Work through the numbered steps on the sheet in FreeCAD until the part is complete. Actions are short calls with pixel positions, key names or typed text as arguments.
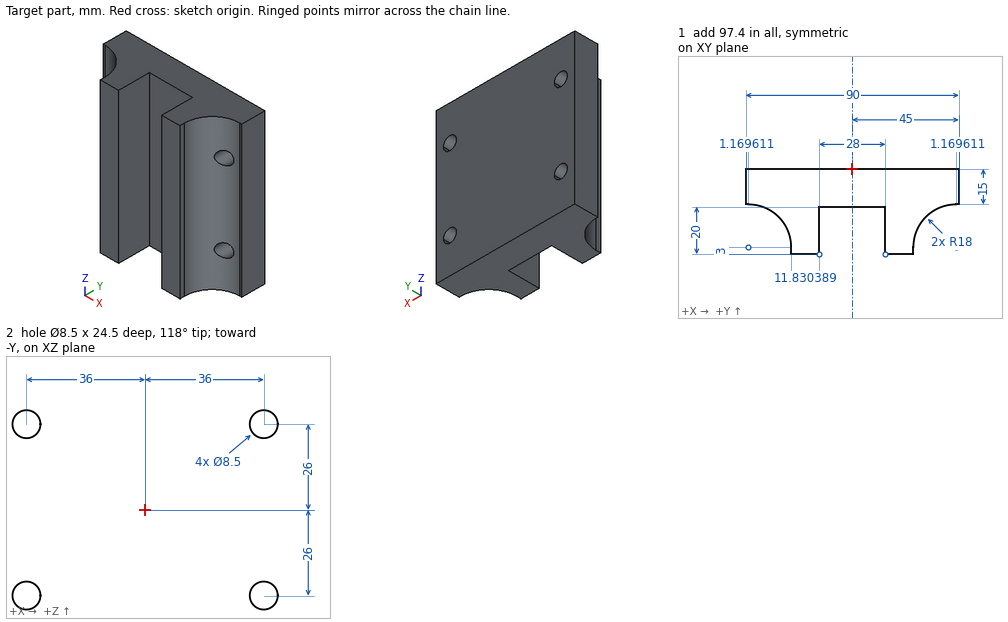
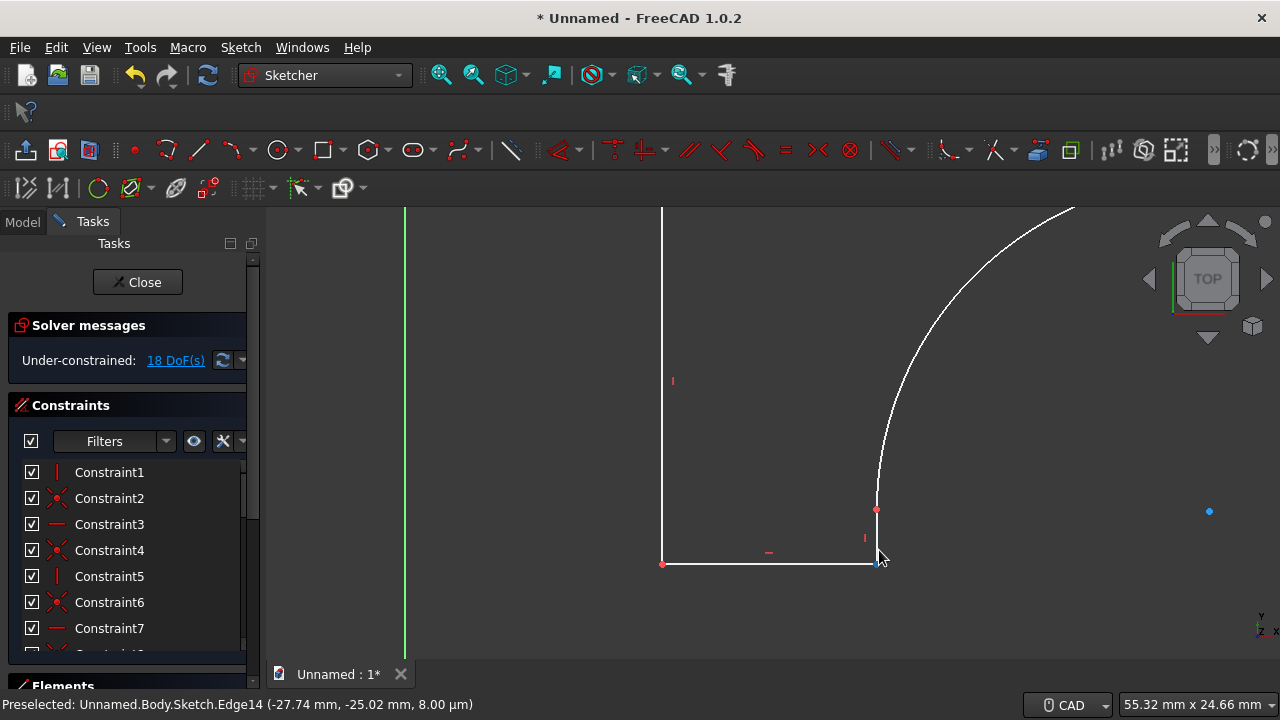
click(877, 548)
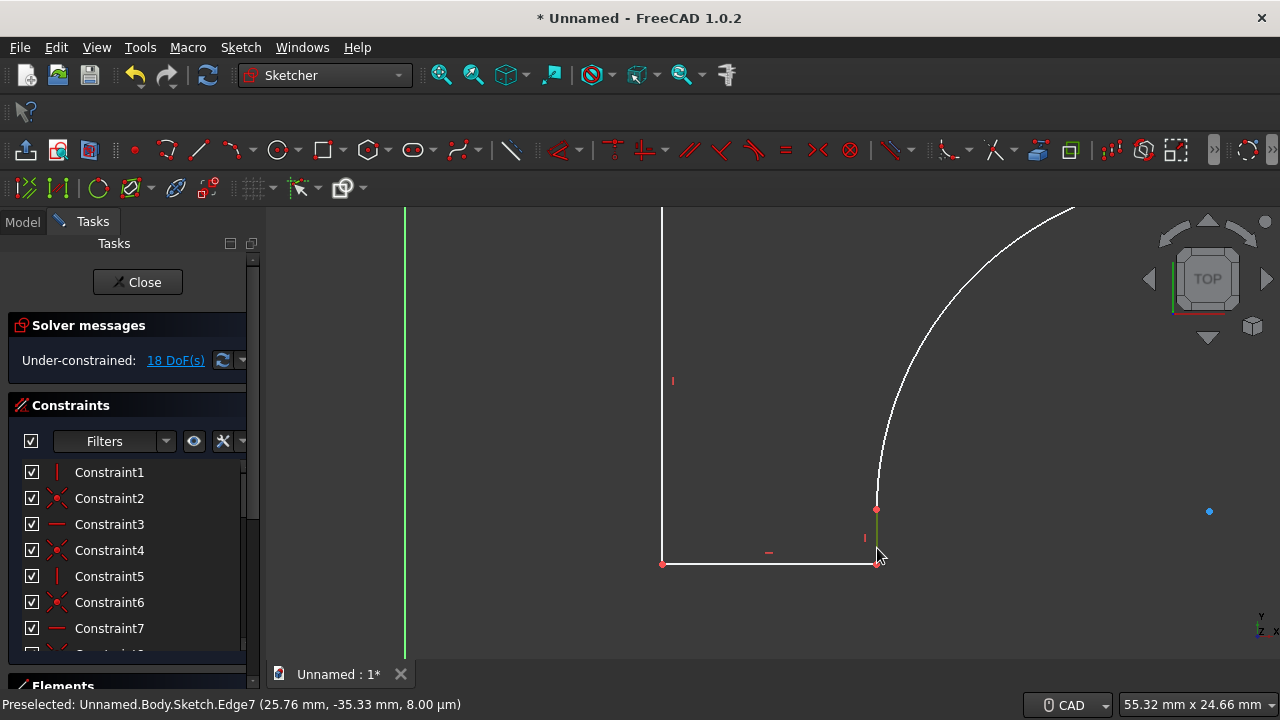
click(913, 360)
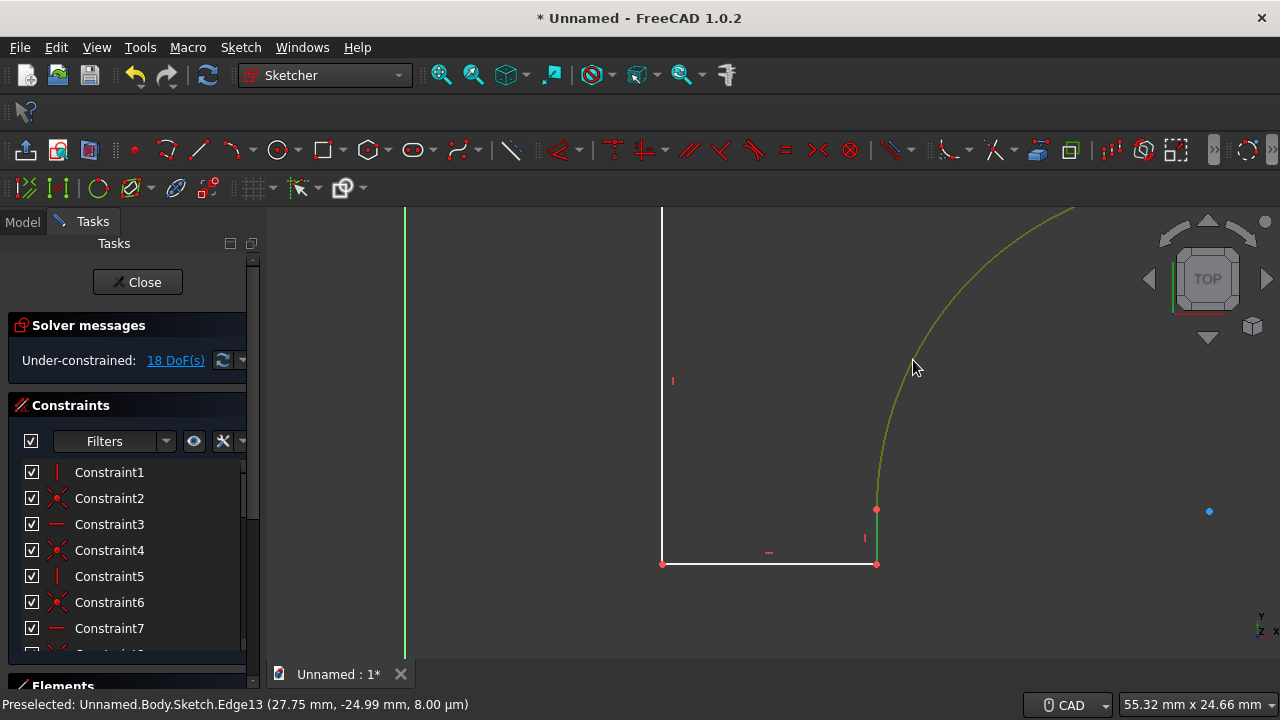
click(754, 150)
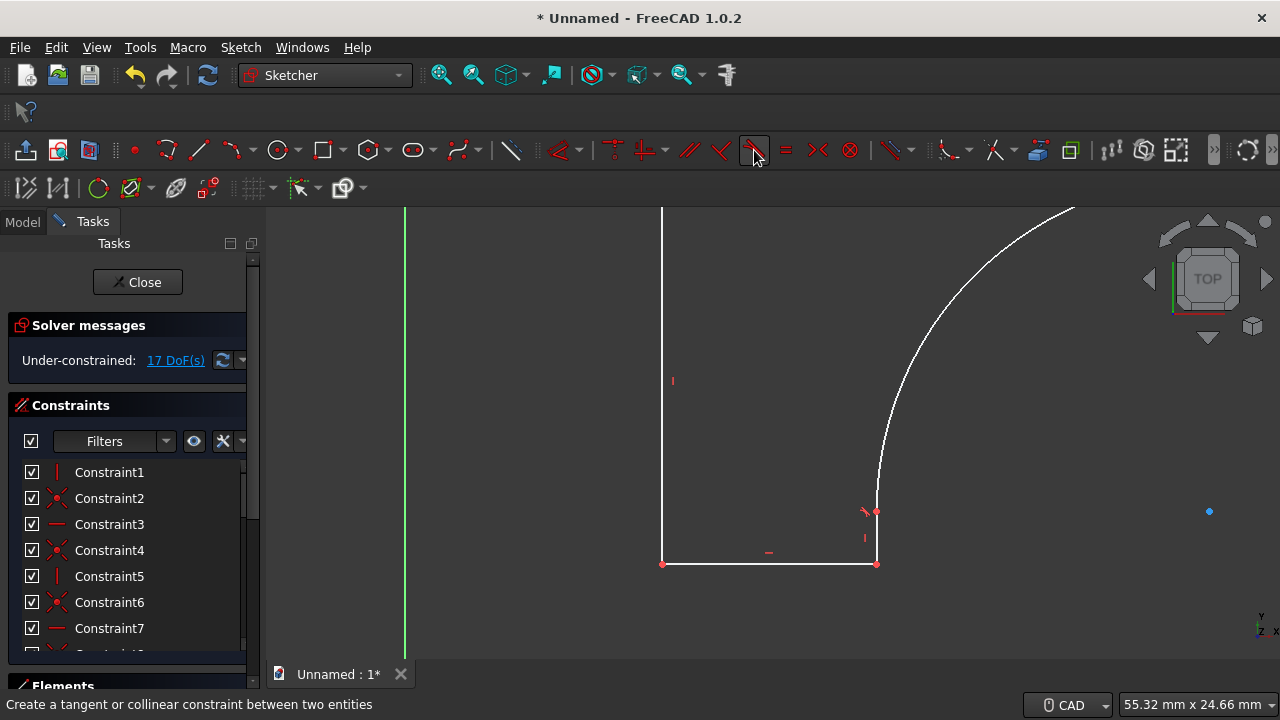
scroll(879, 550, down, 5)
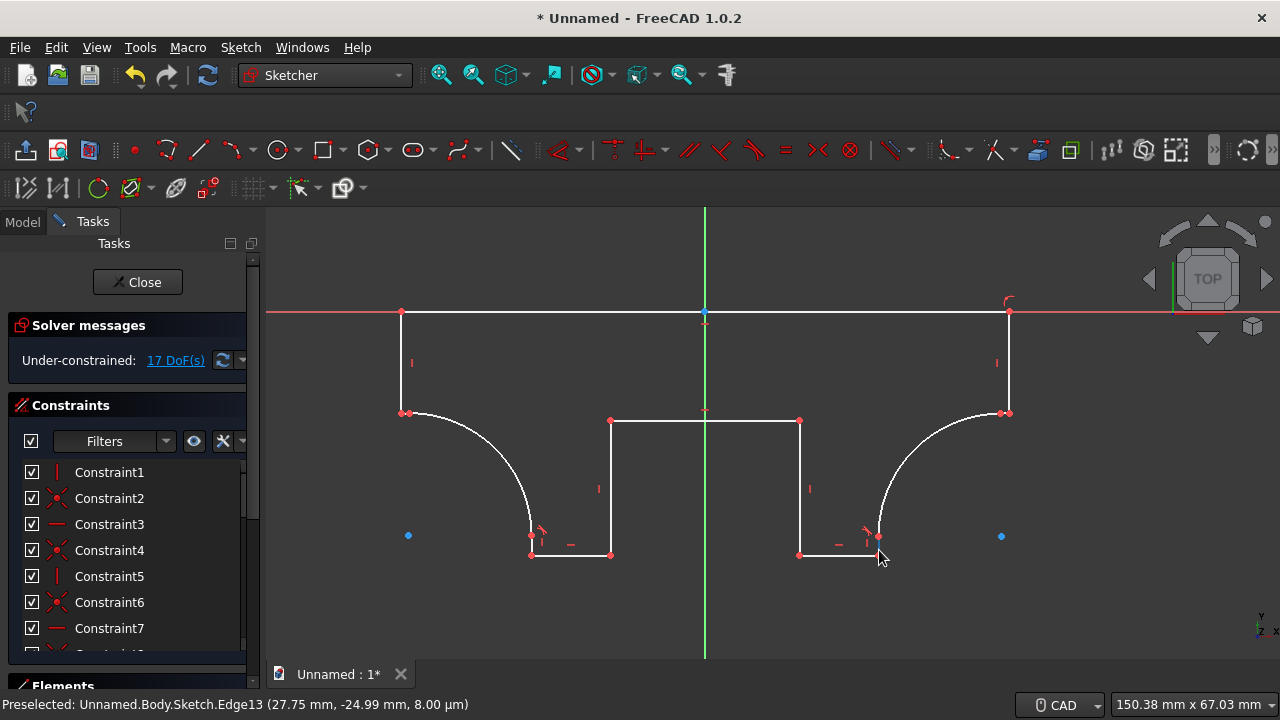
scroll(1004, 413, up, 8)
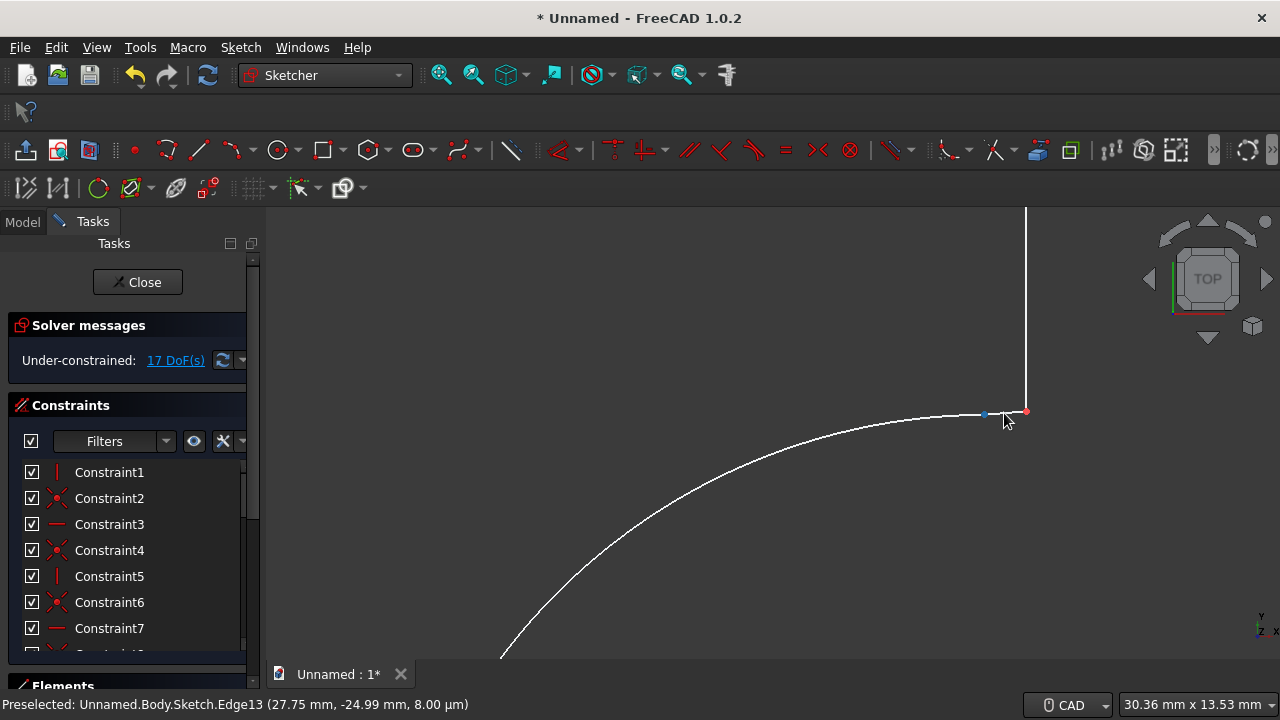
click(1001, 413)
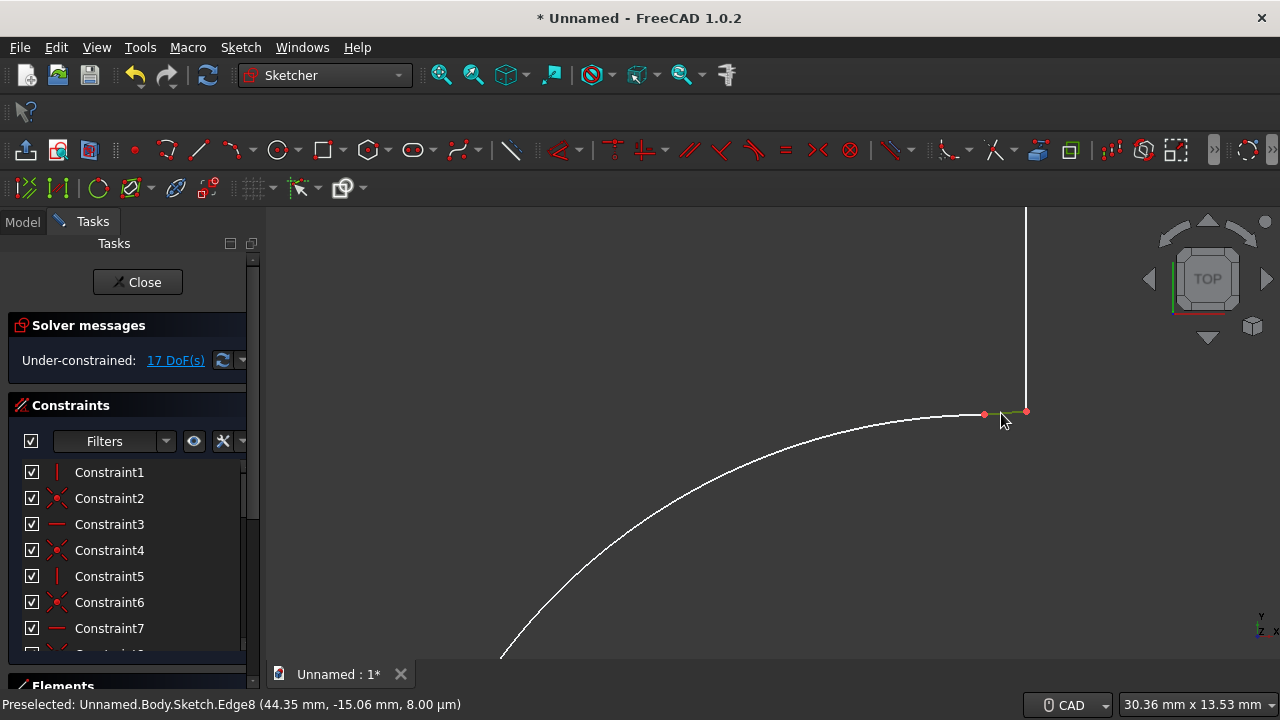
scroll(1004, 413, down, 8)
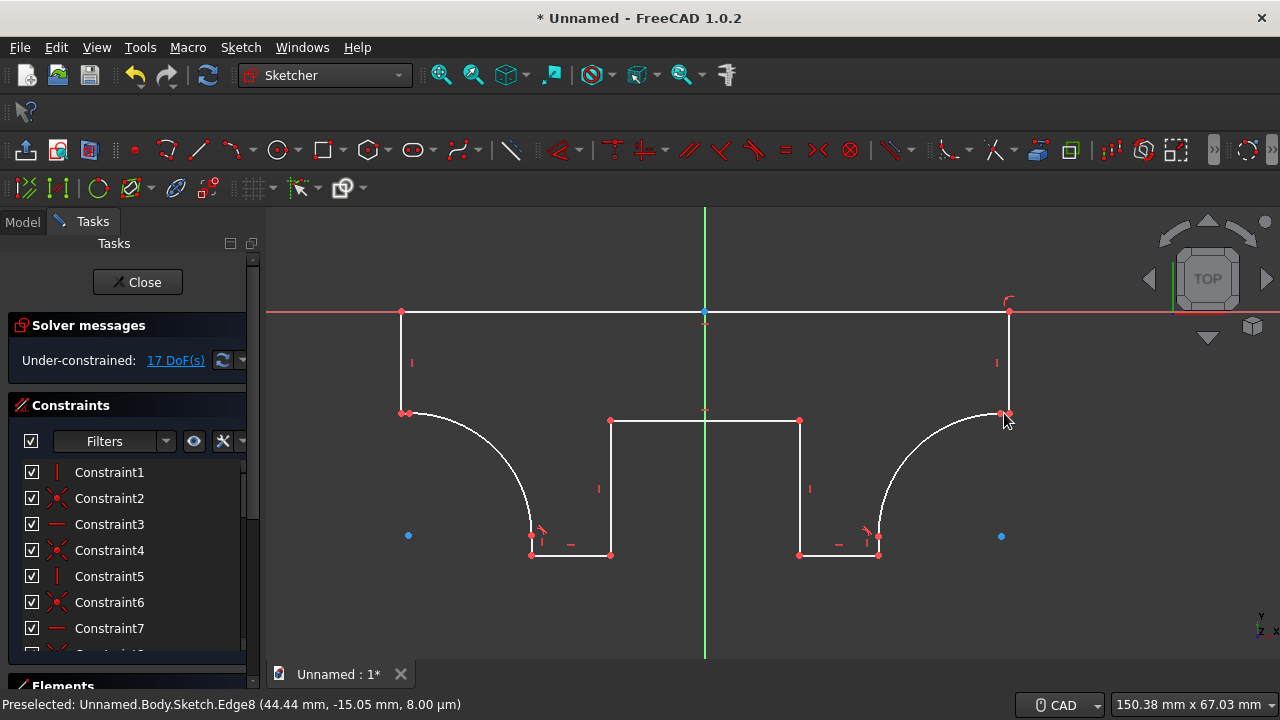
click(945, 427)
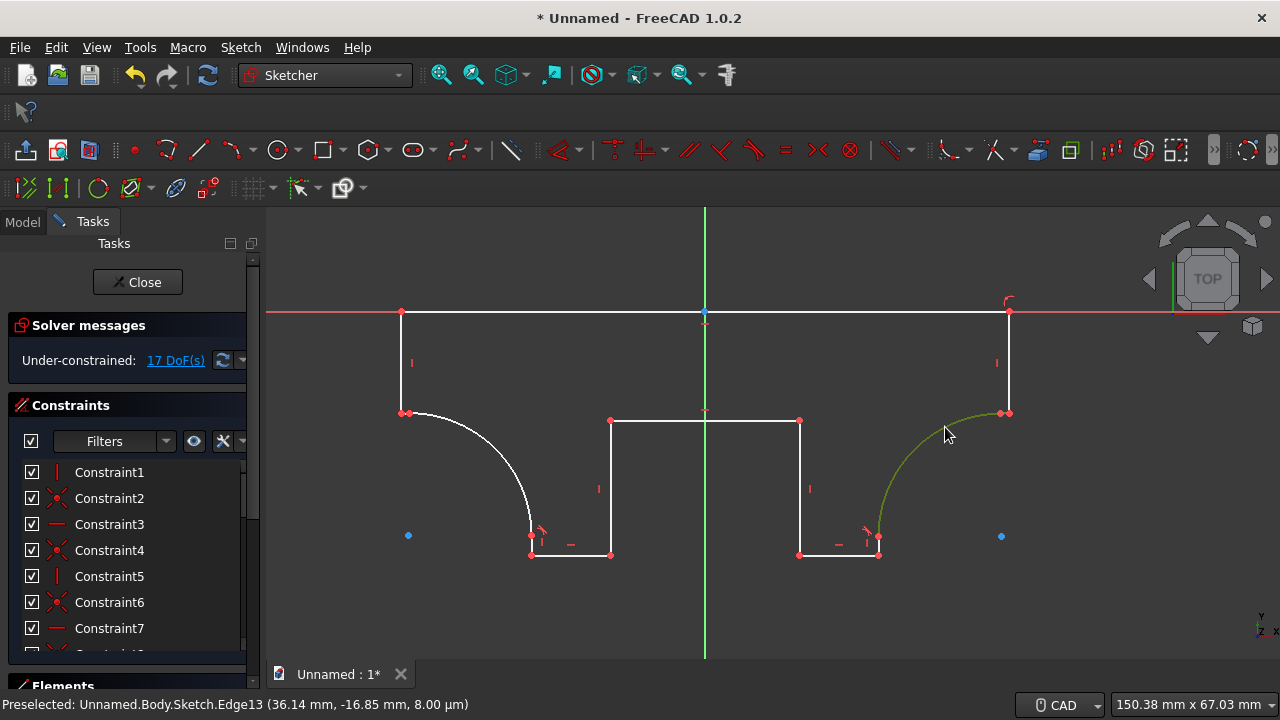
click(754, 150)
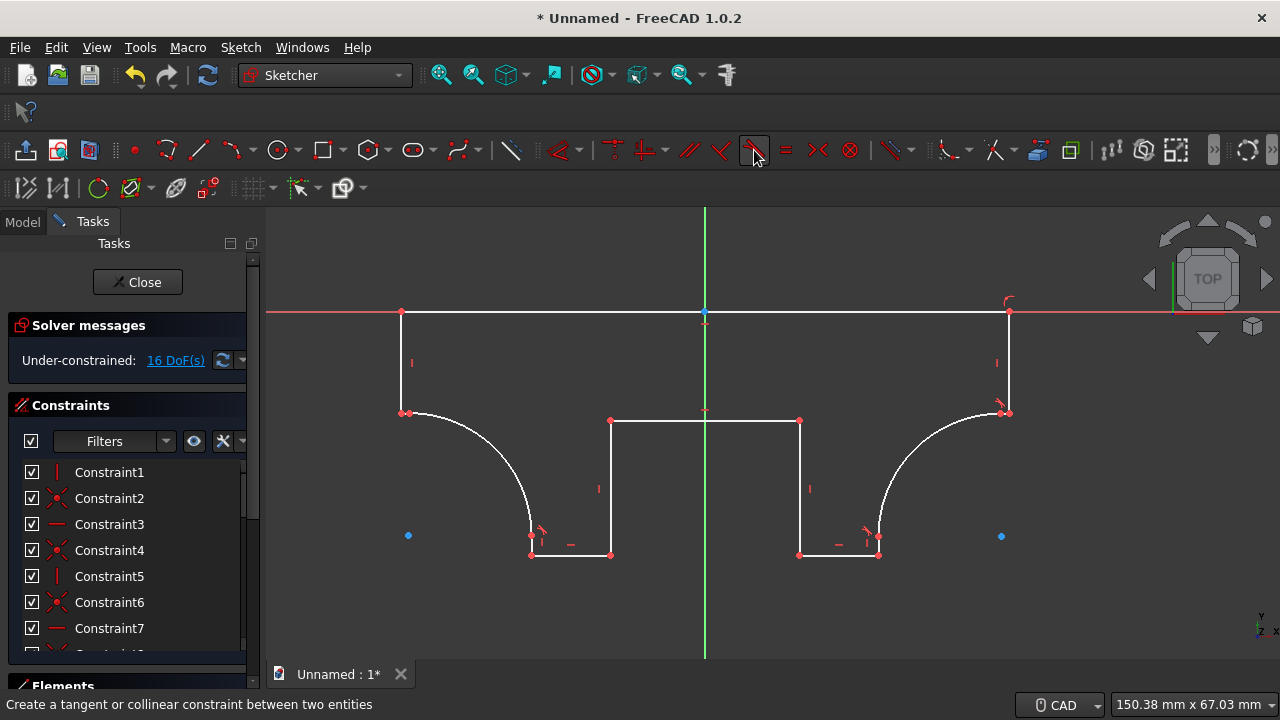
scroll(405, 414, up, 6)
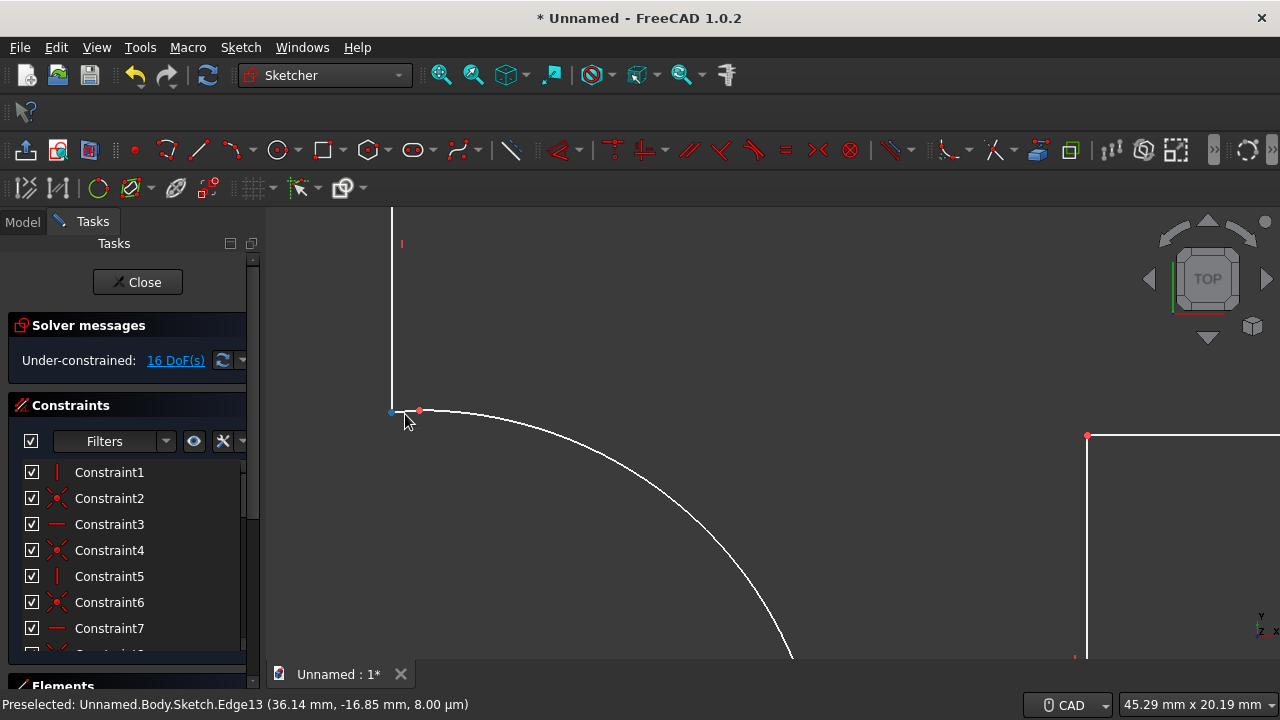
click(406, 411)